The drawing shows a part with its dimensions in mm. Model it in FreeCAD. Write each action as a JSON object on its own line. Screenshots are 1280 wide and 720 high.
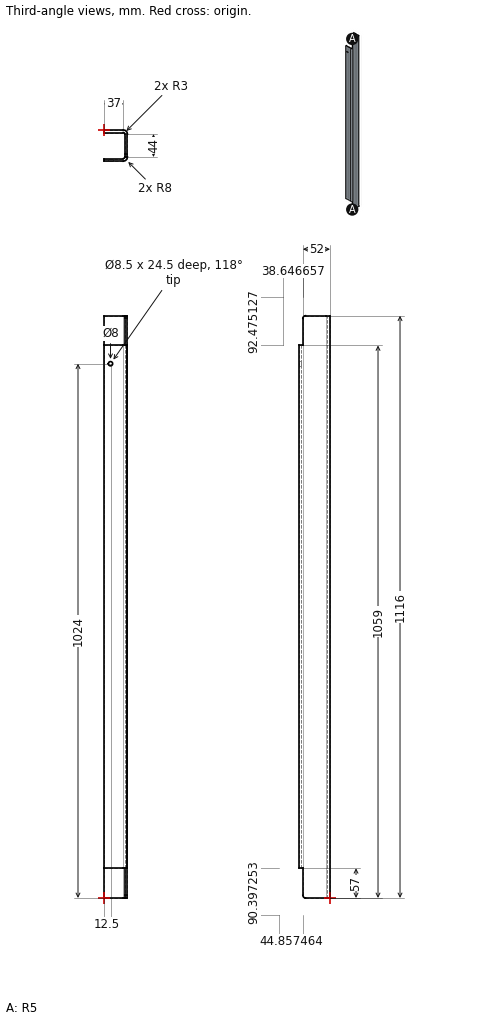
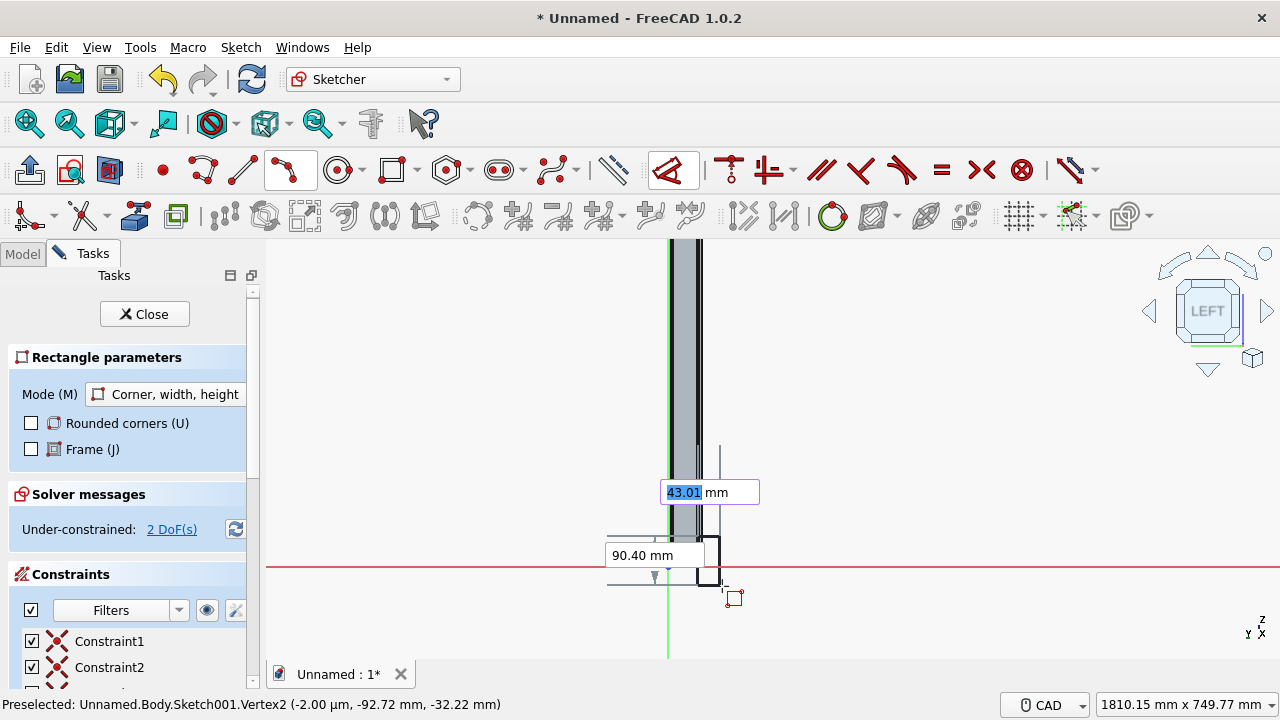
{"action": "type", "text": "44.857464"}
{"action": "key", "text": "Tab"}
{"action": "type", "text": "90.397253"}
{"action": "key", "text": "Return"}
{"action": "key", "text": "Escape"}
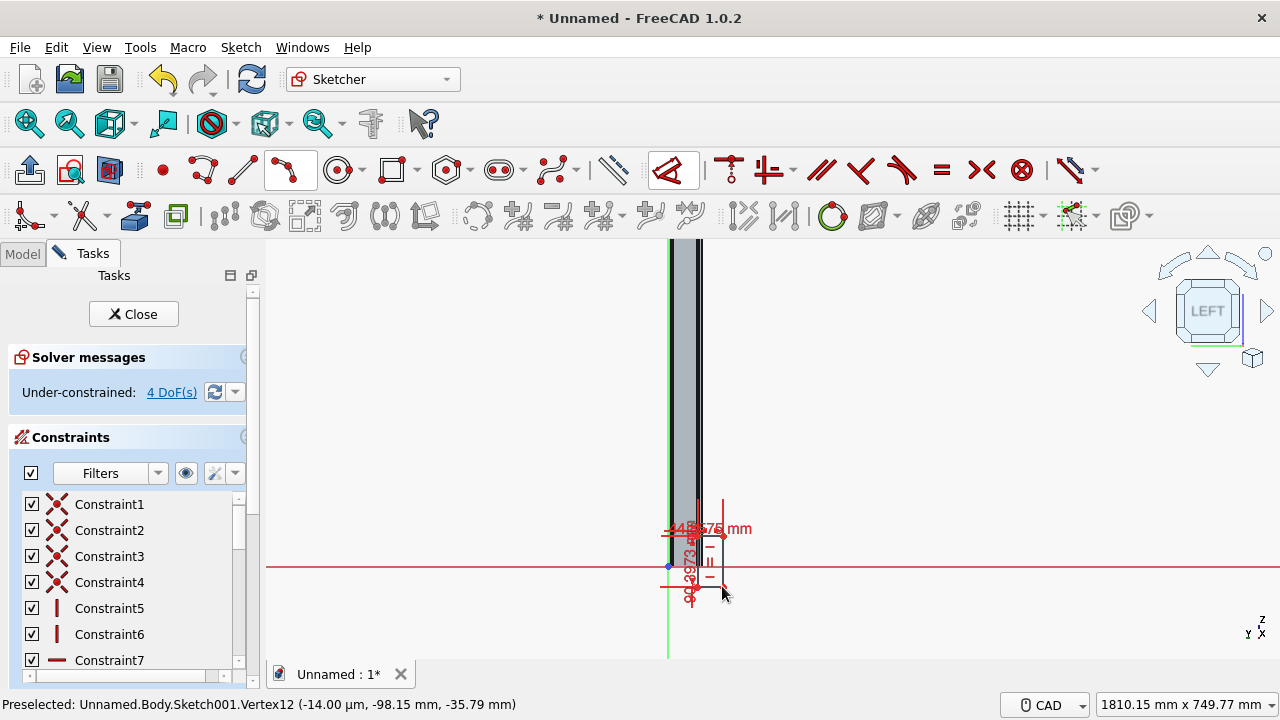
{"action": "left_click", "coordinate": [668, 170]}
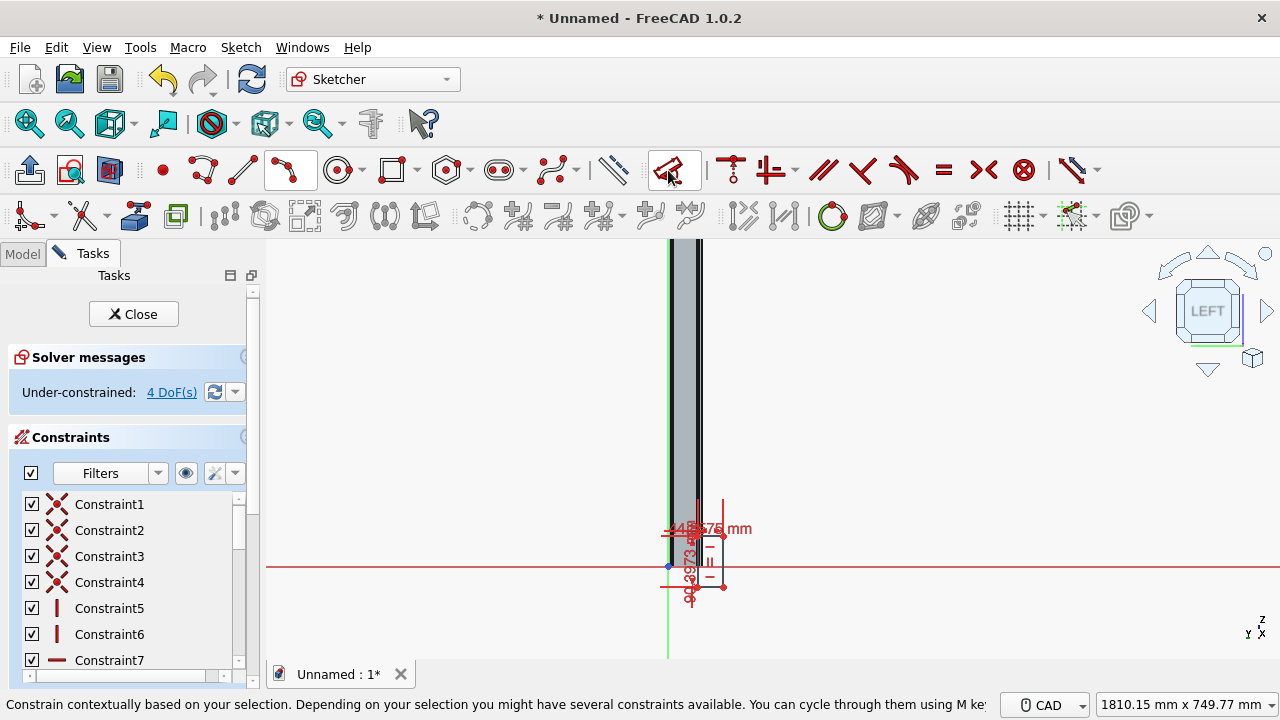
{"action": "scroll", "coordinate": [710, 563], "scroll_direction": "down", "scroll_amount": 5}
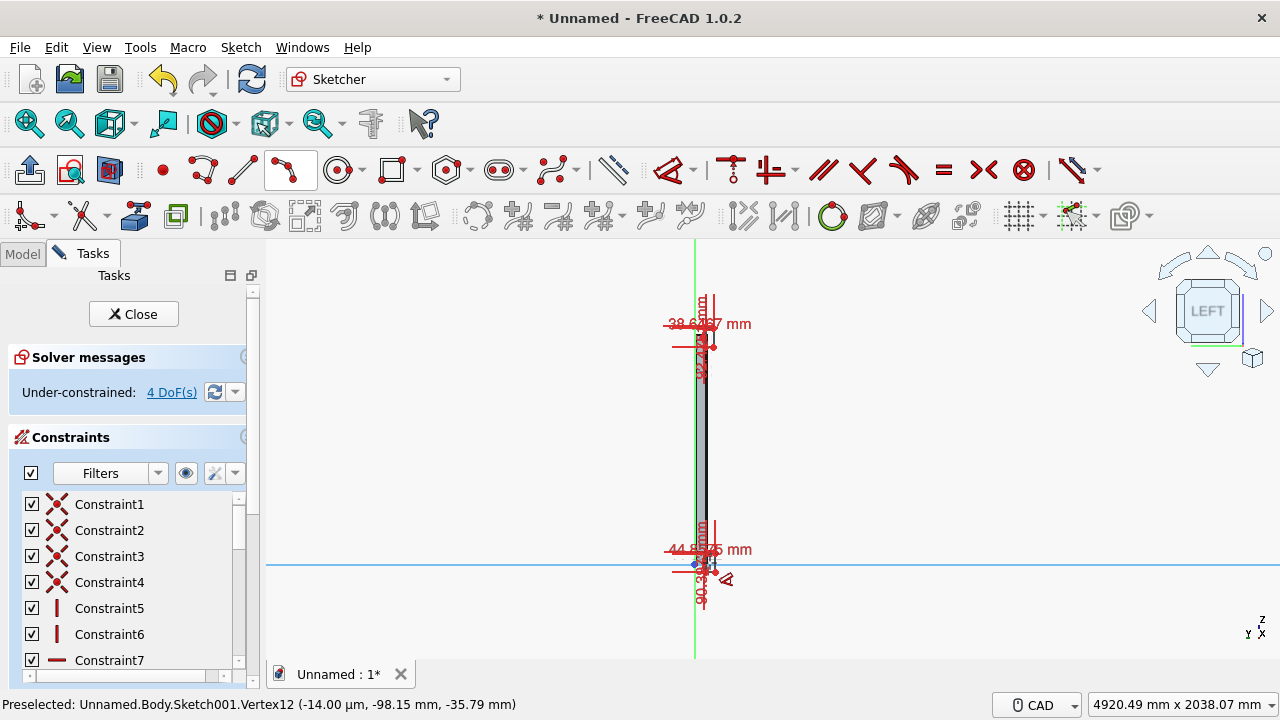
{"action": "scroll", "coordinate": [706, 328], "scroll_direction": "up", "scroll_amount": 7}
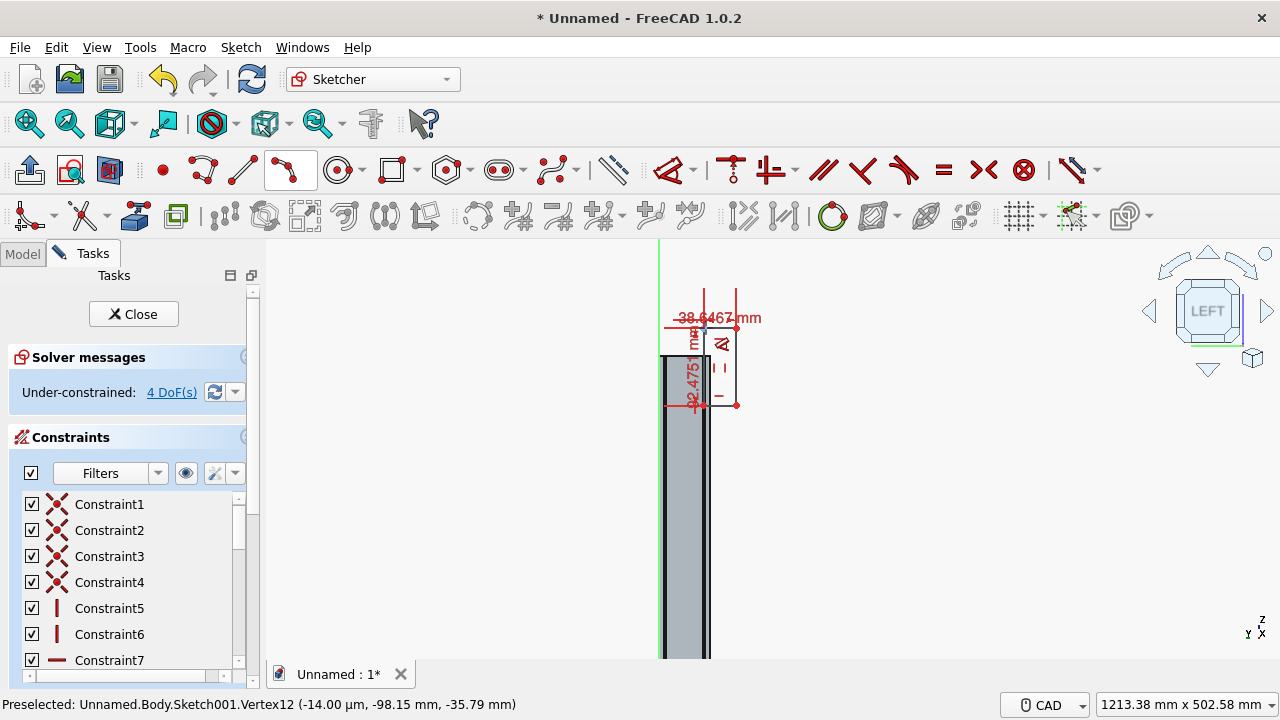
{"action": "left_click", "coordinate": [704, 328]}
{"action": "left_click", "coordinate": [682, 294]}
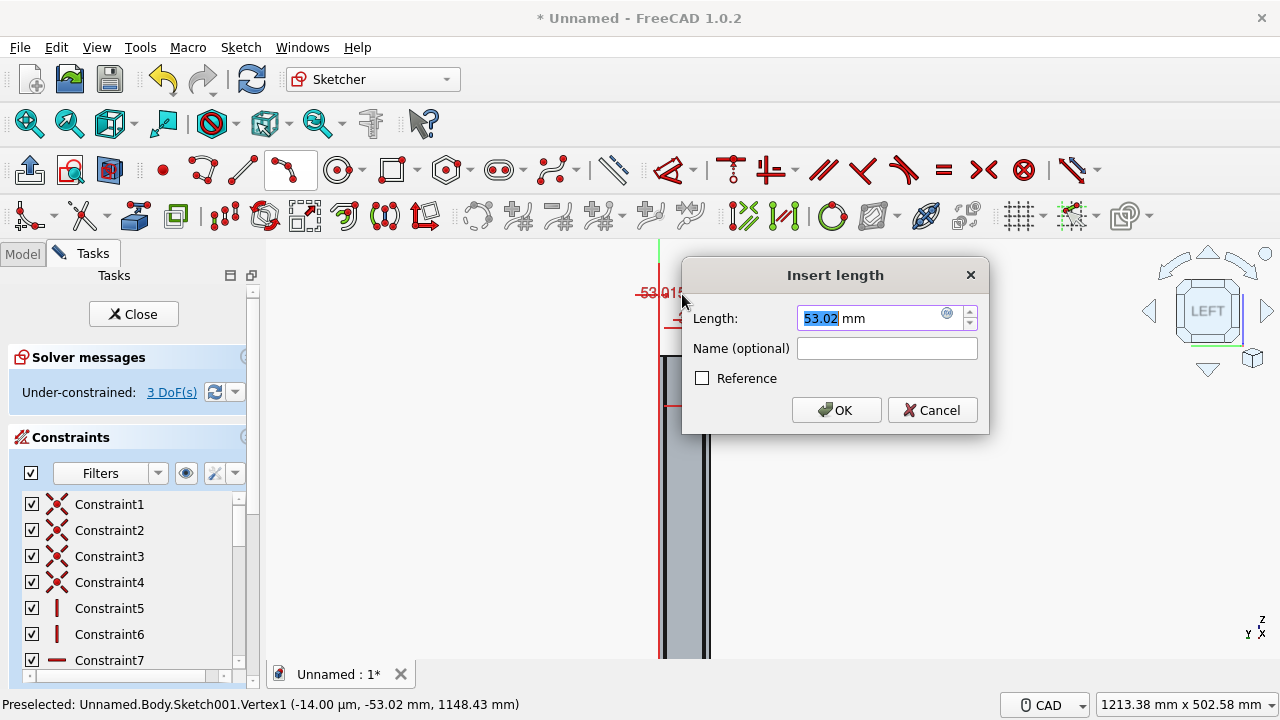
{"action": "type", "text": "52"}
{"action": "key", "text": "Return"}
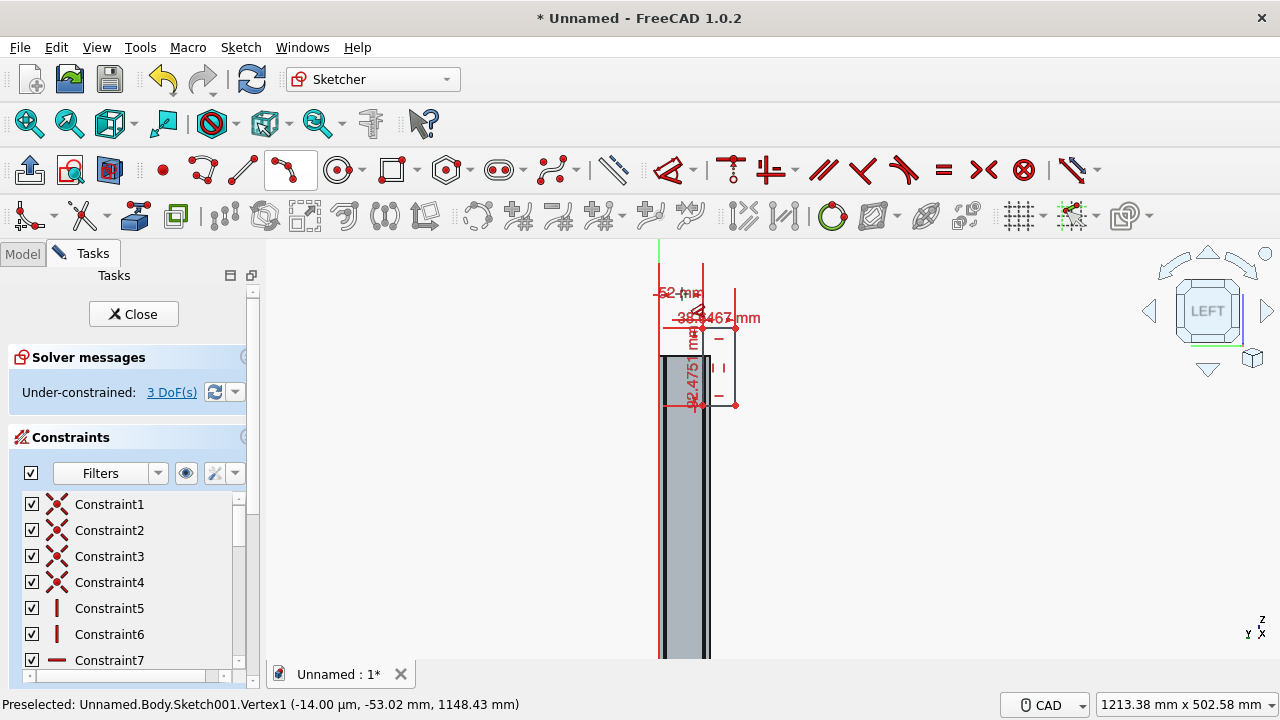
{"action": "scroll", "coordinate": [706, 327], "scroll_direction": "down", "scroll_amount": 7}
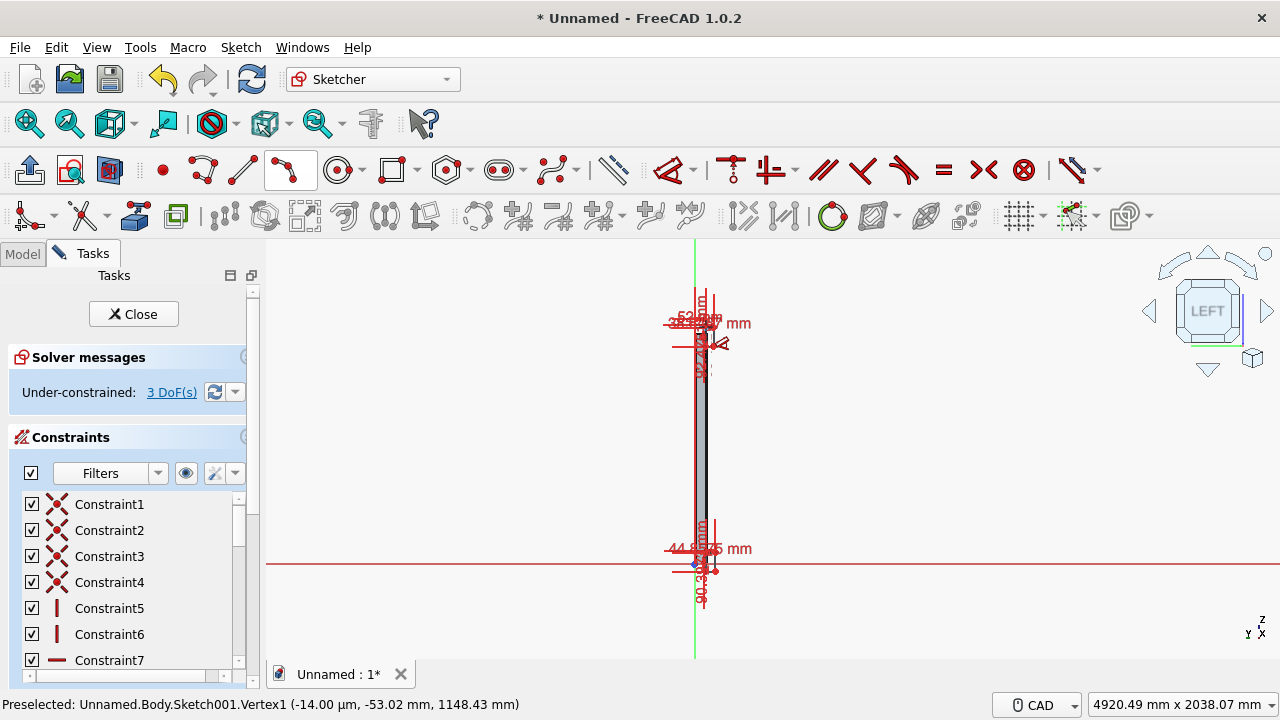
{"action": "scroll", "coordinate": [706, 553], "scroll_direction": "up", "scroll_amount": 7}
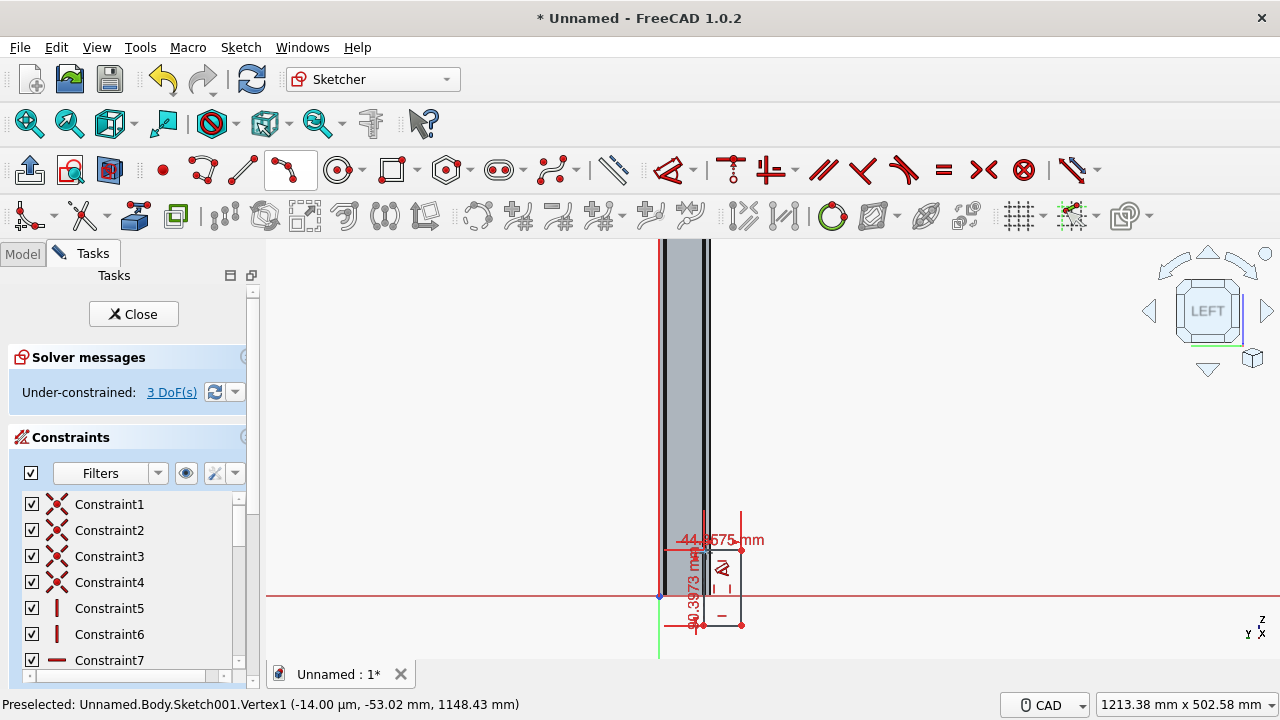
{"action": "left_click", "coordinate": [704, 550]}
{"action": "left_click", "coordinate": [682, 630]}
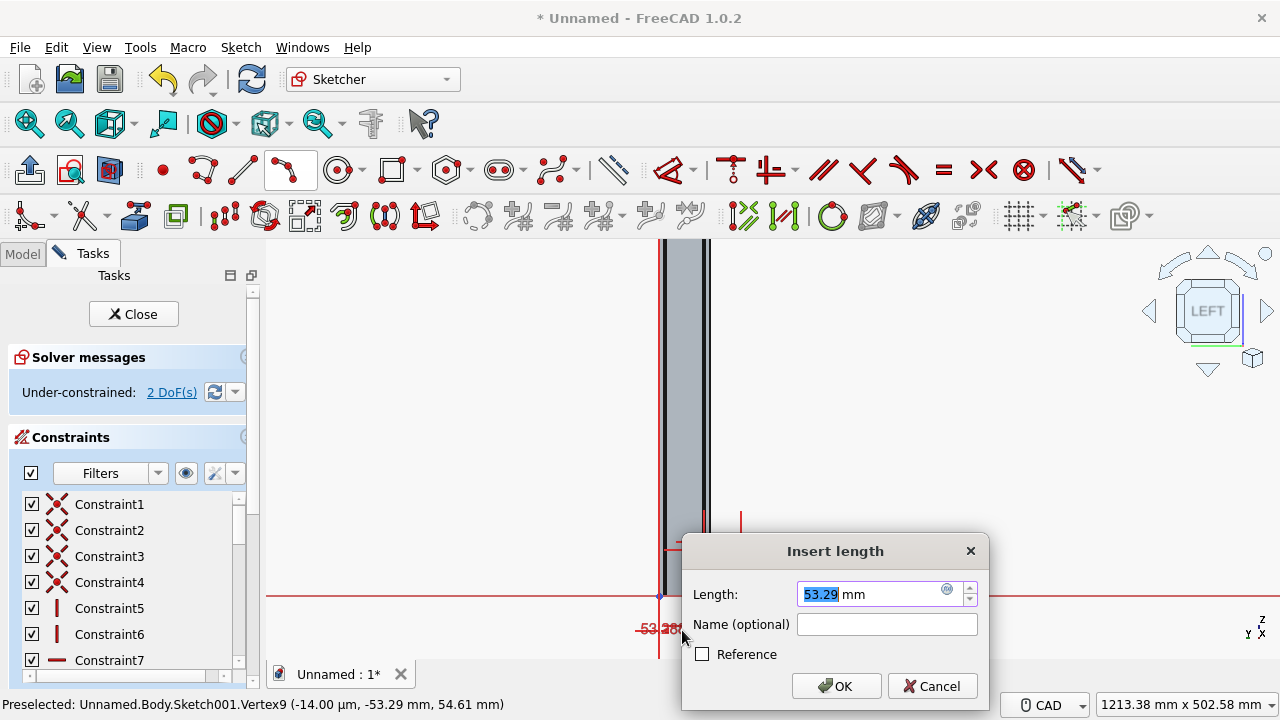
{"action": "type", "text": "52"}
{"action": "key", "text": "Return"}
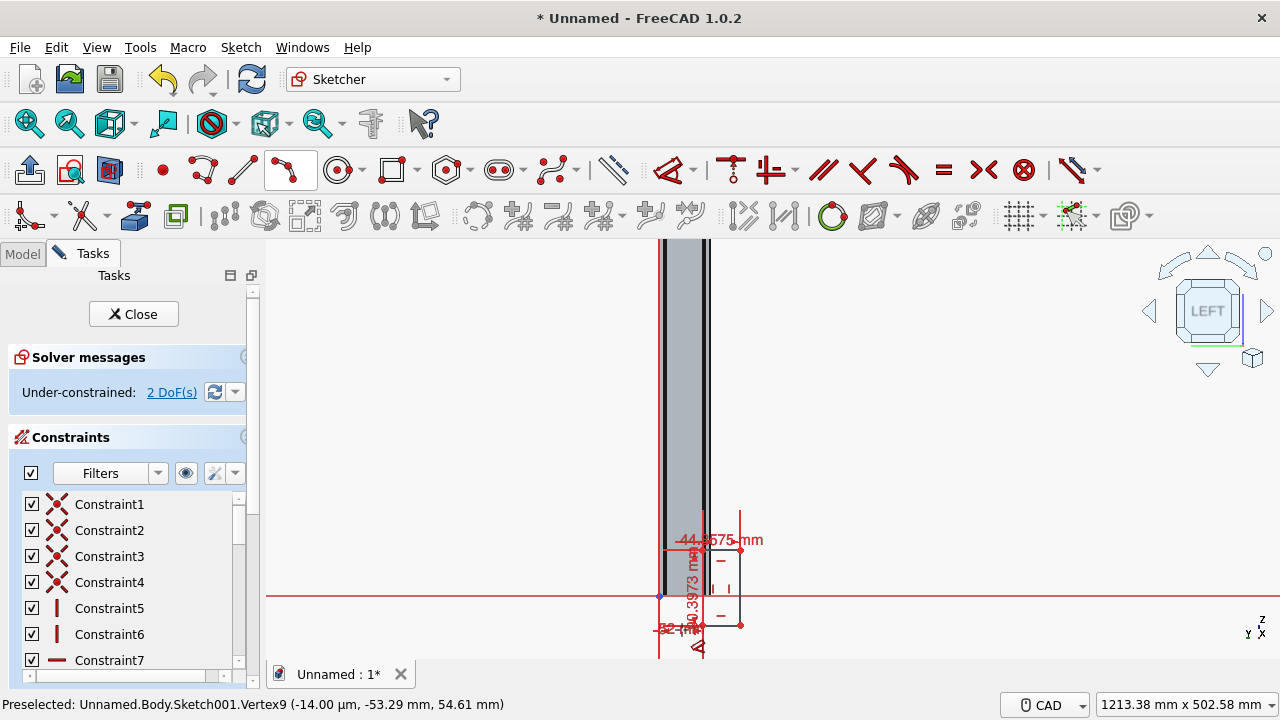
{"action": "left_click", "coordinate": [703, 550]}
{"action": "left_click", "coordinate": [625, 573]}